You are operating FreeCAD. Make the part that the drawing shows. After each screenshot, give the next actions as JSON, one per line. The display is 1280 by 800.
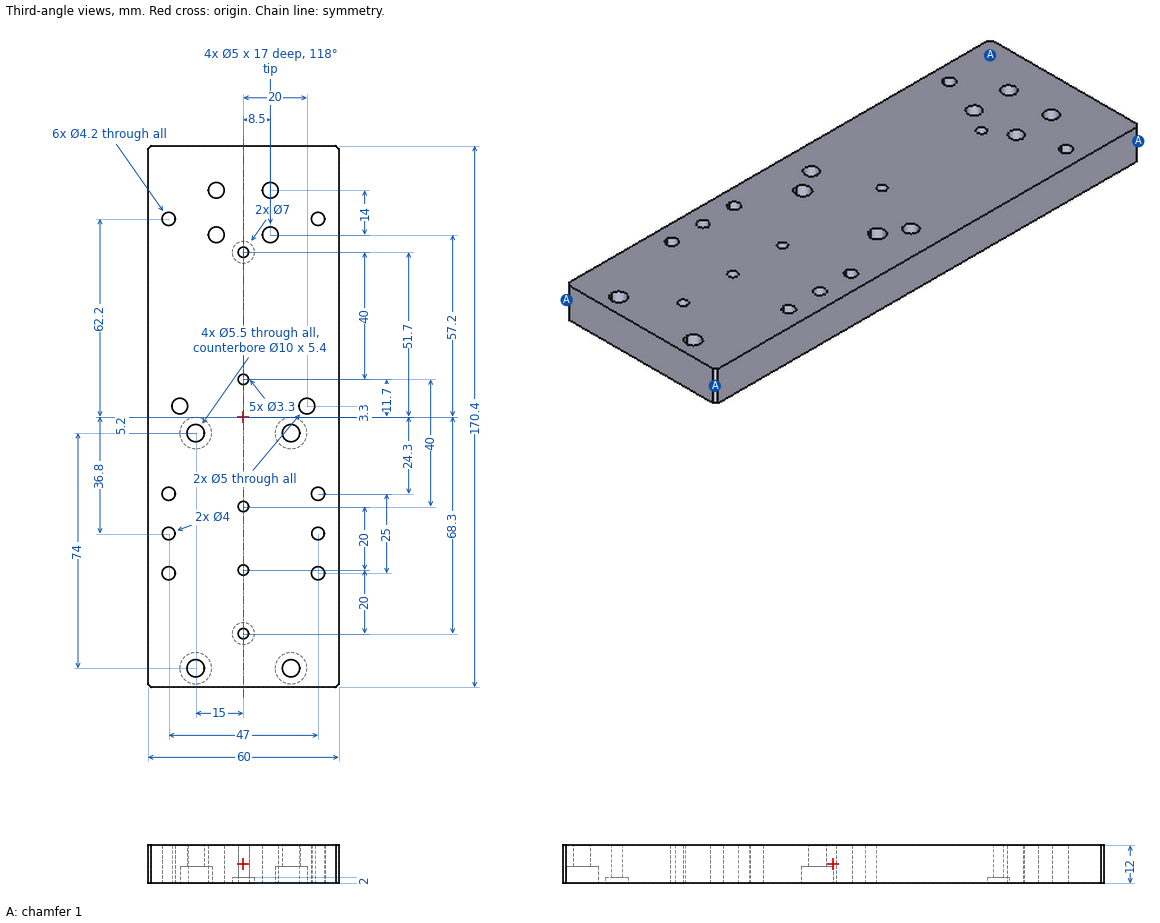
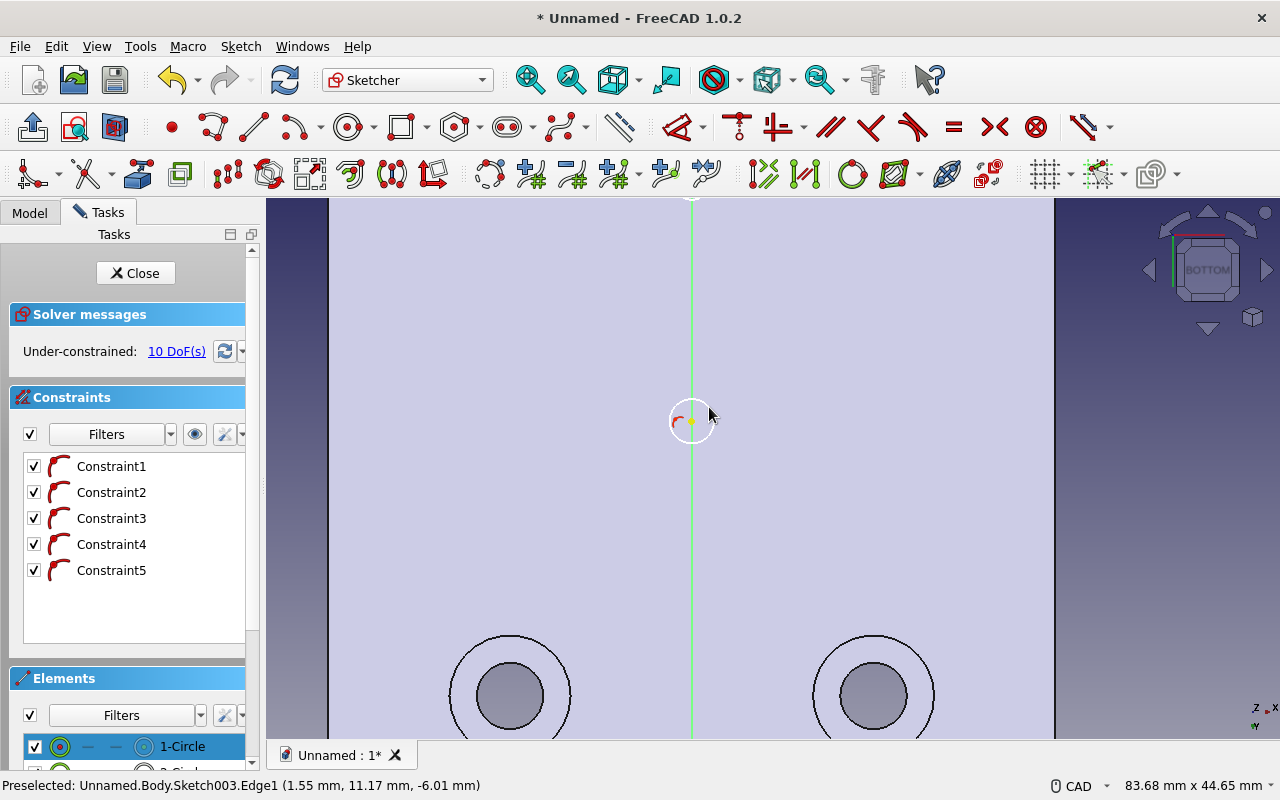
{"action": "left_click", "coordinate": [707, 406]}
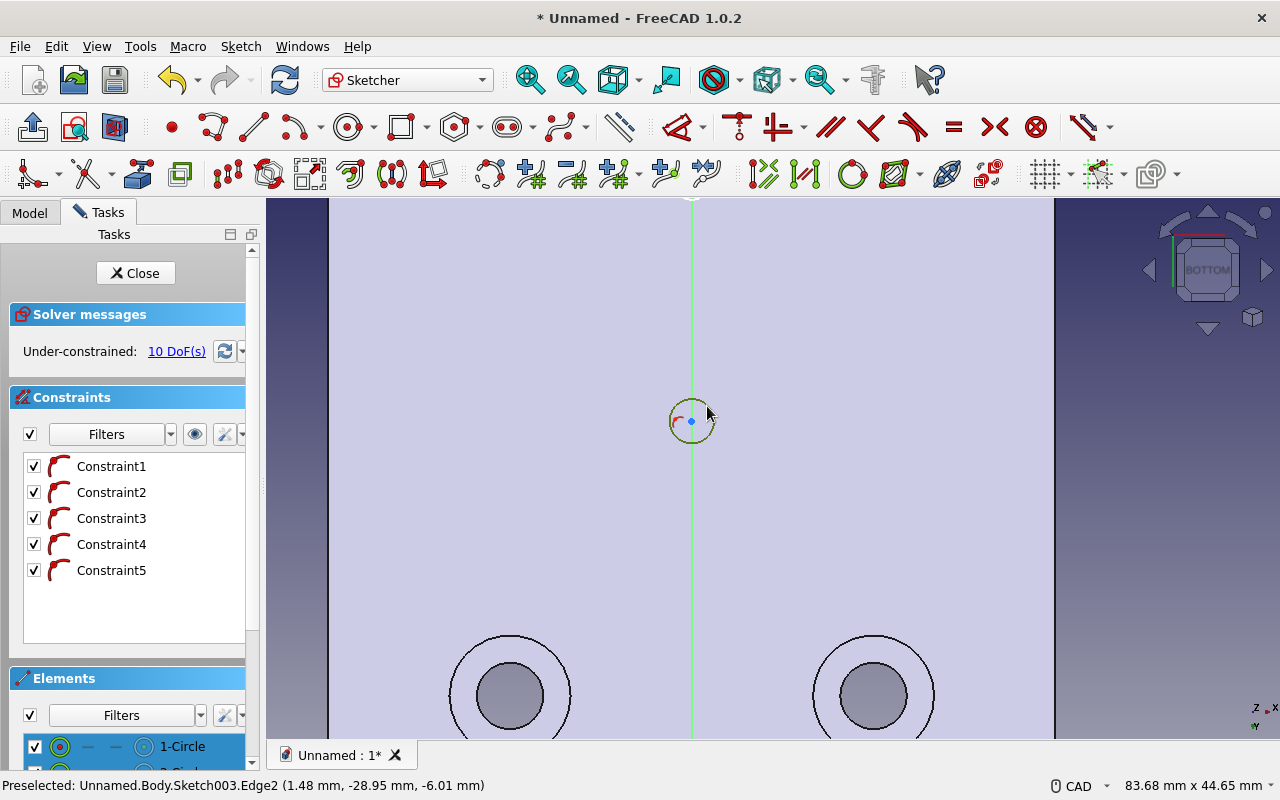
{"action": "scroll", "coordinate": [709, 406], "scroll_direction": "down", "scroll_amount": 7}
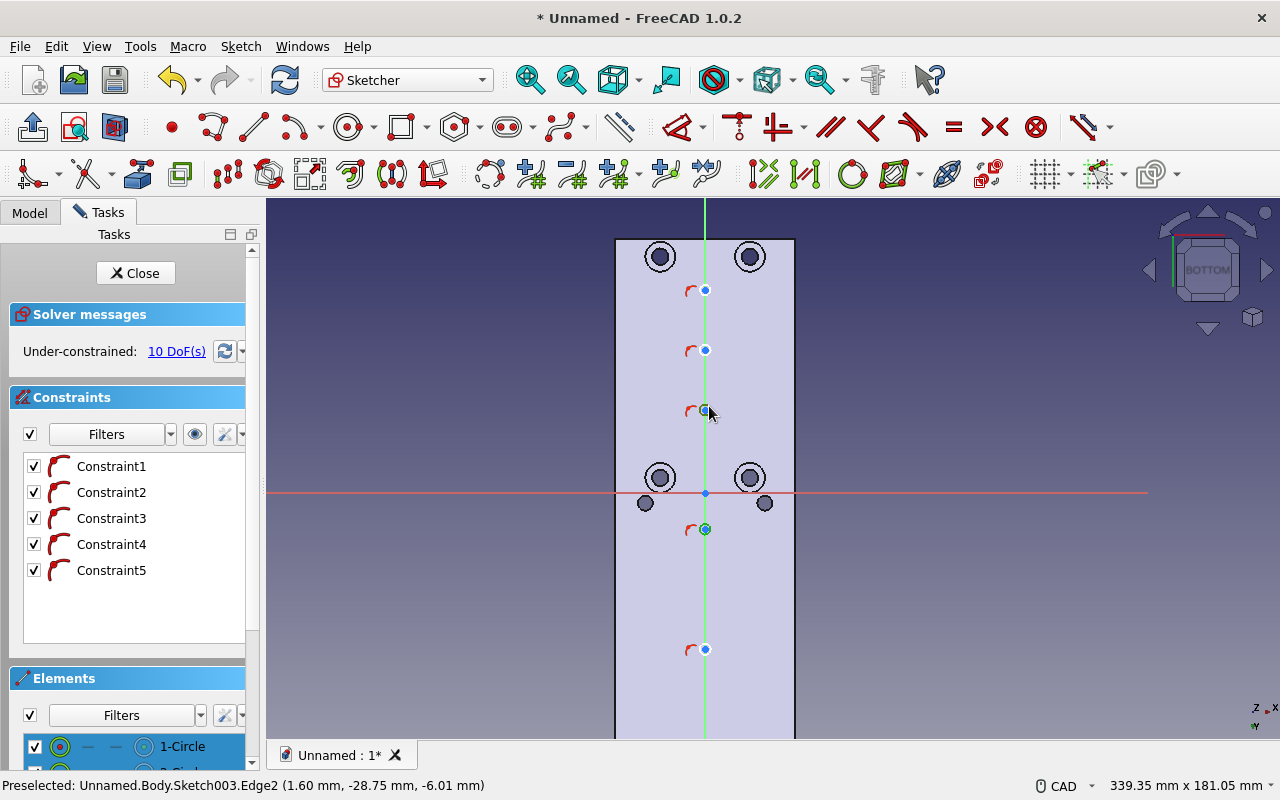
{"action": "scroll", "coordinate": [709, 346], "scroll_direction": "up", "scroll_amount": 7}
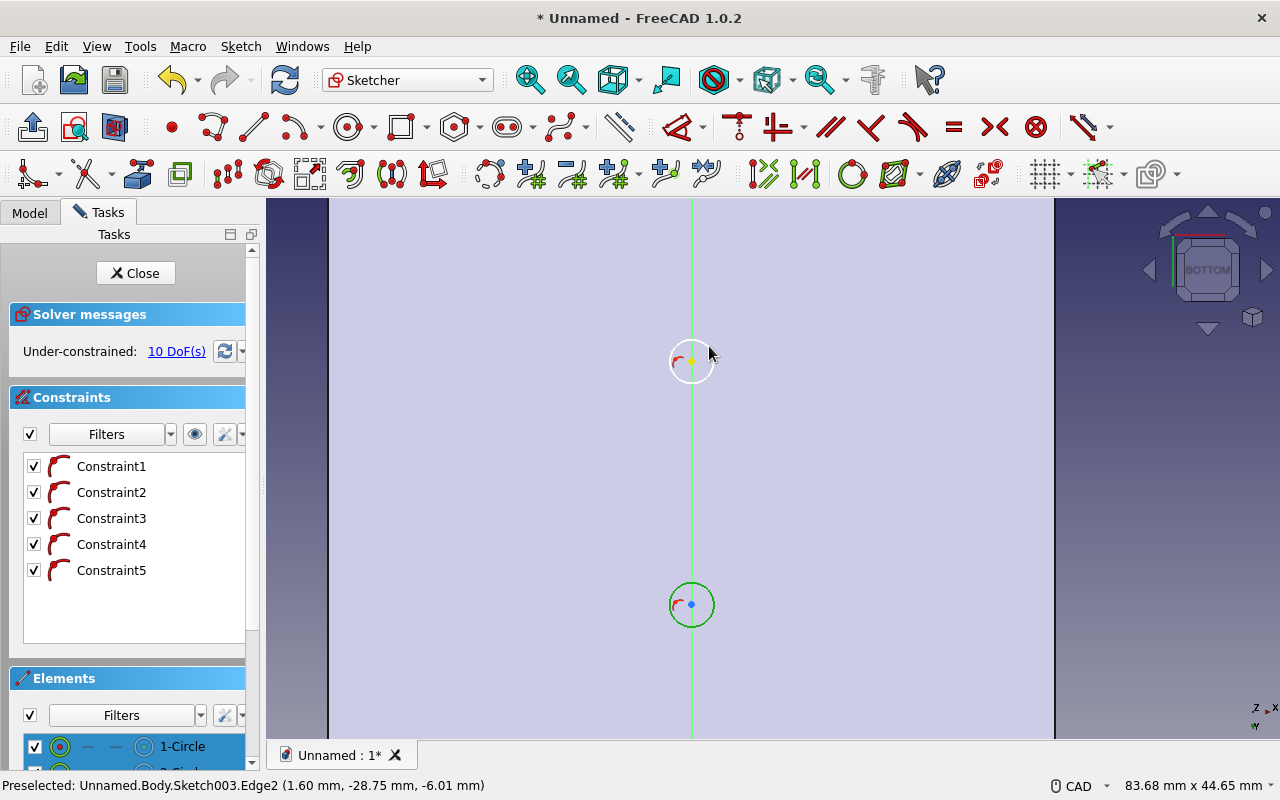
{"action": "left_click", "coordinate": [707, 346]}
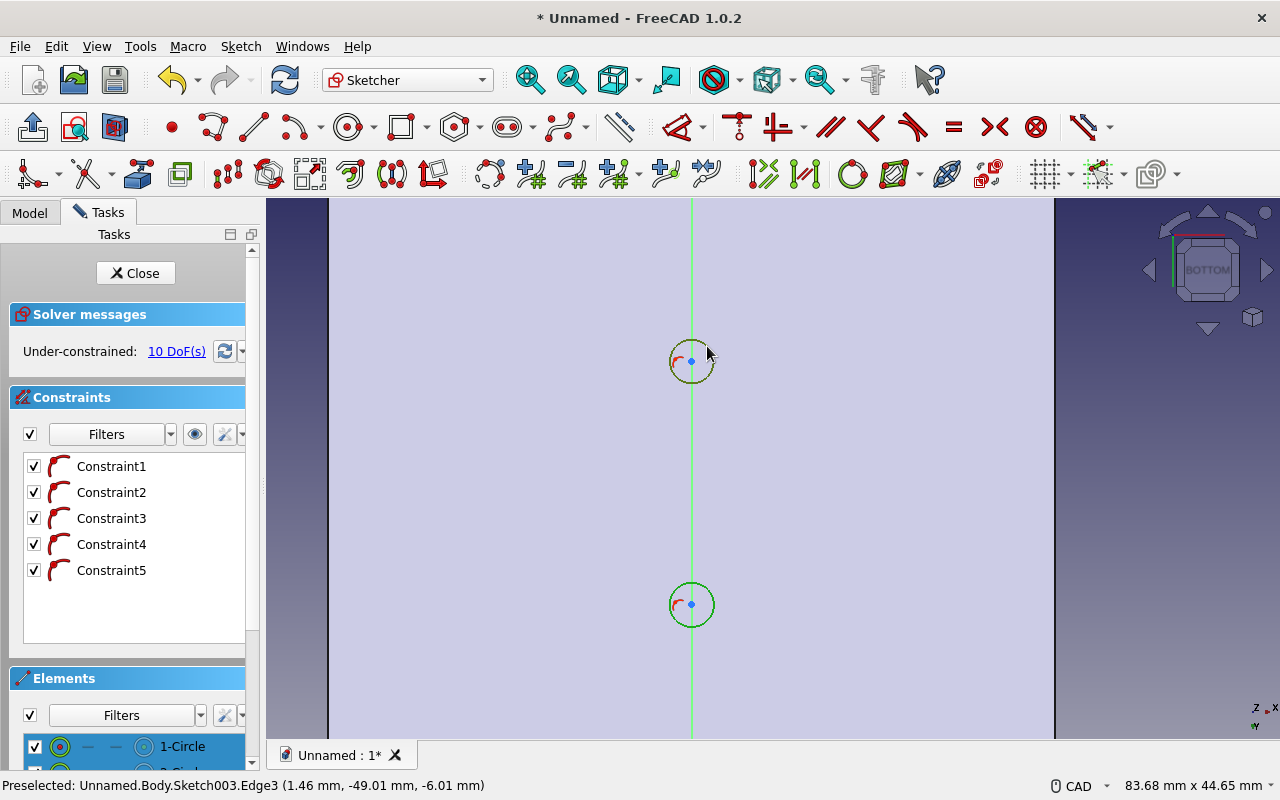
{"action": "scroll", "coordinate": [709, 346], "scroll_direction": "down", "scroll_amount": 7}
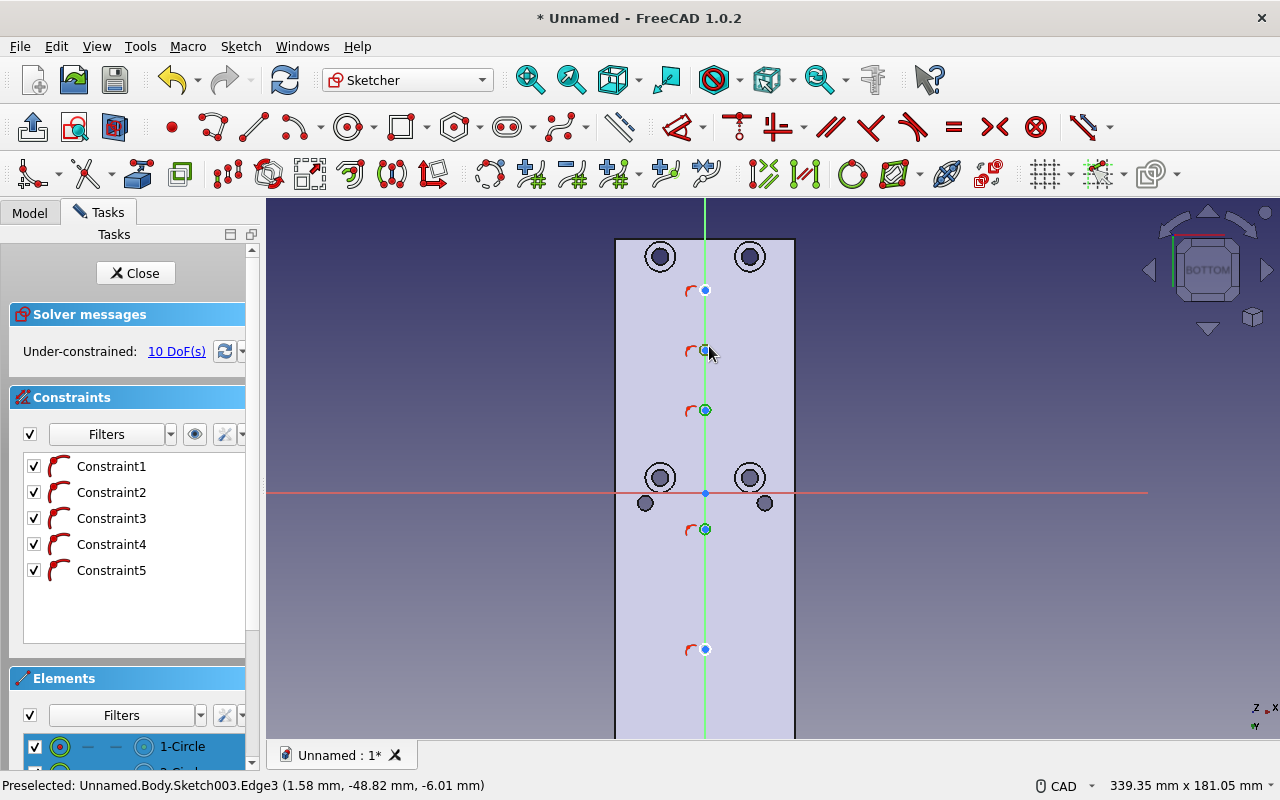
{"action": "scroll", "coordinate": [709, 286], "scroll_direction": "up", "scroll_amount": 7}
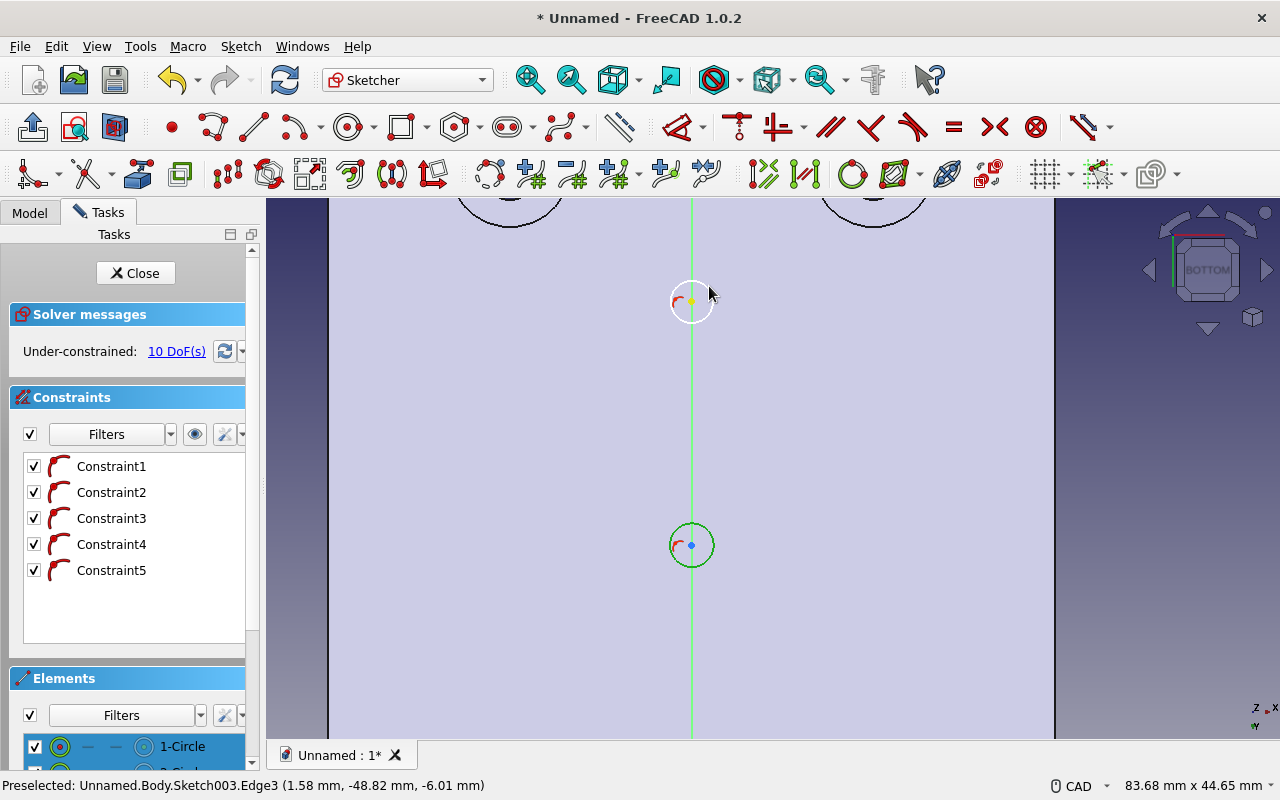
{"action": "left_click", "coordinate": [707, 287]}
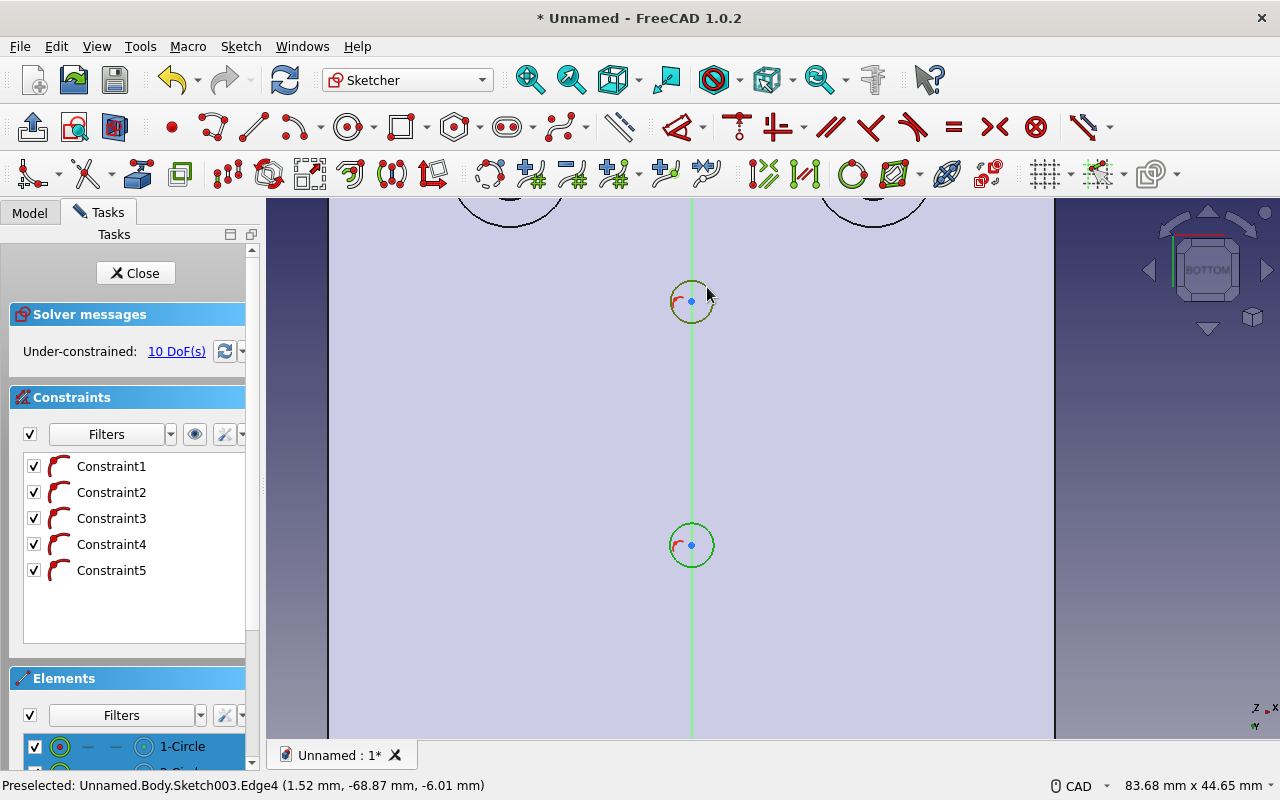
{"action": "scroll", "coordinate": [709, 286], "scroll_direction": "down", "scroll_amount": 7}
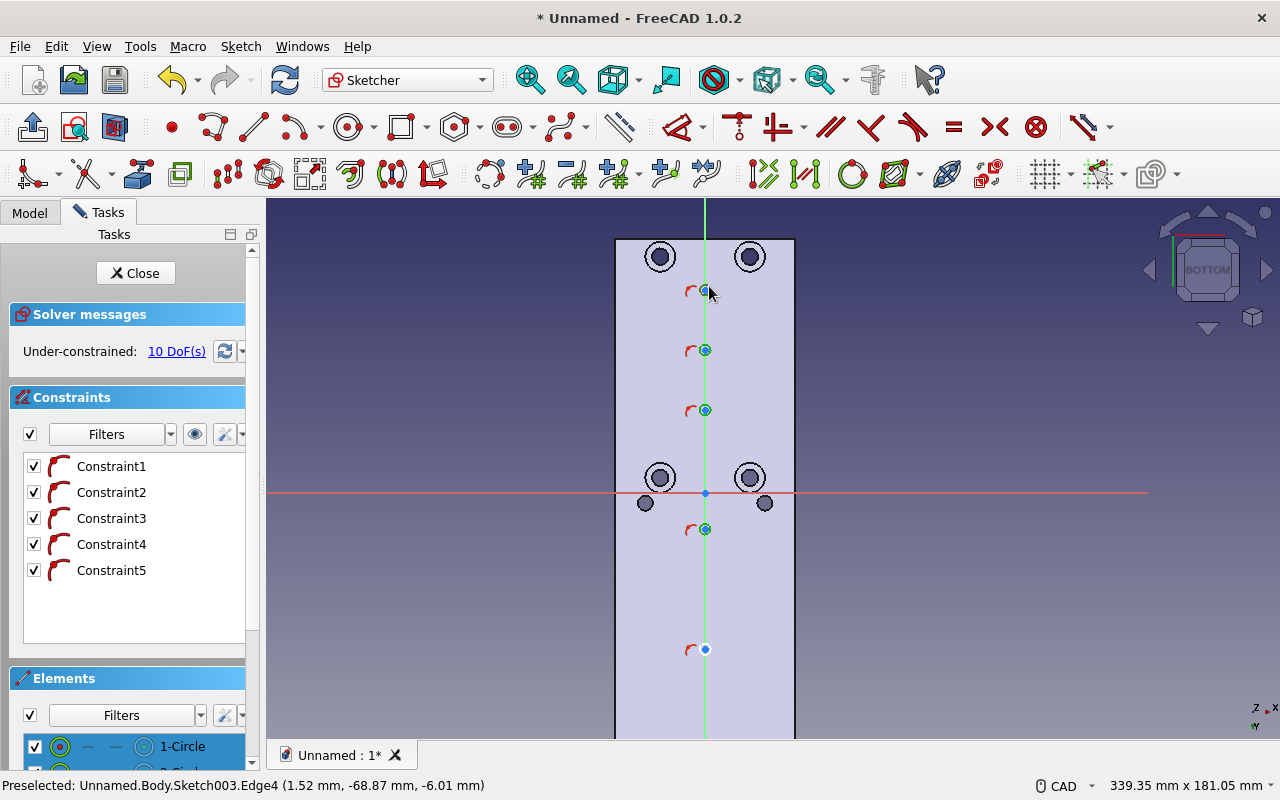
{"action": "scroll", "coordinate": [709, 645], "scroll_direction": "up", "scroll_amount": 7}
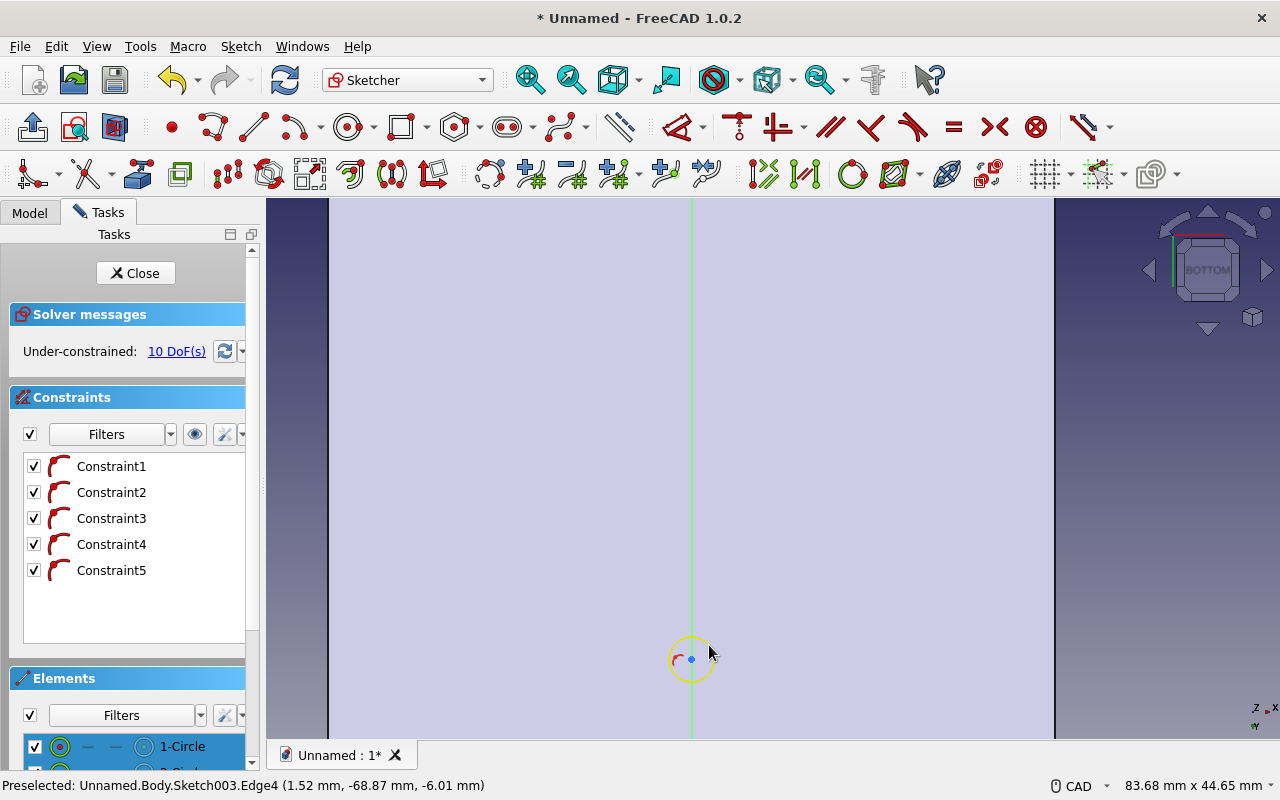
{"action": "left_click", "coordinate": [708, 644]}